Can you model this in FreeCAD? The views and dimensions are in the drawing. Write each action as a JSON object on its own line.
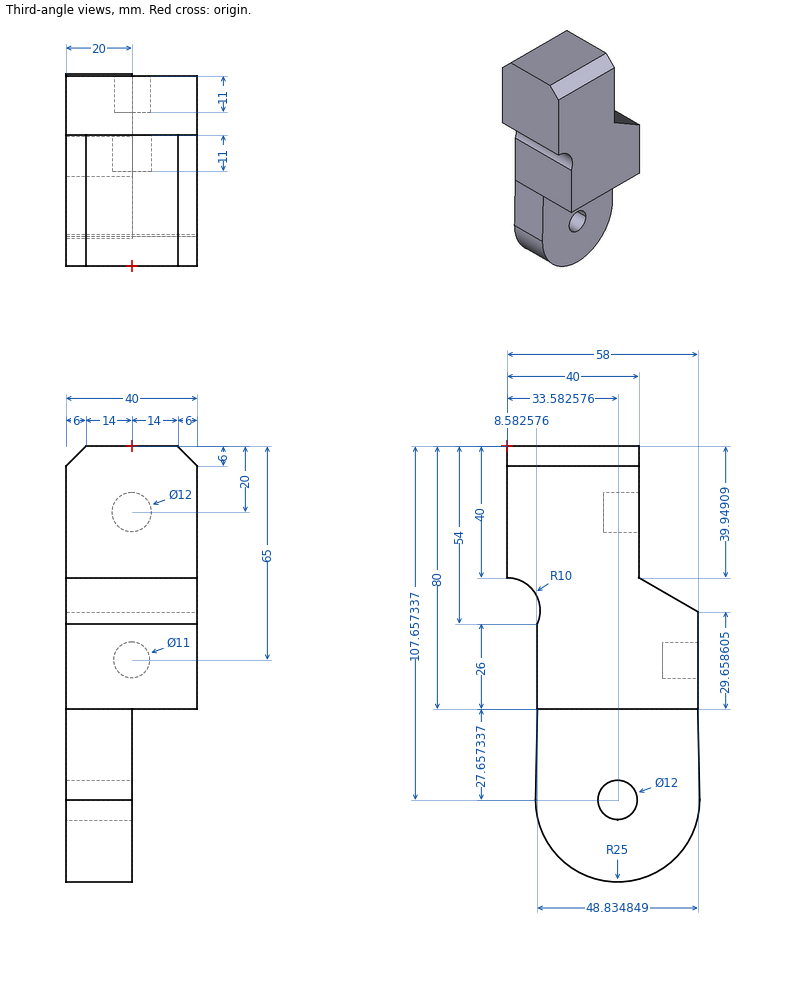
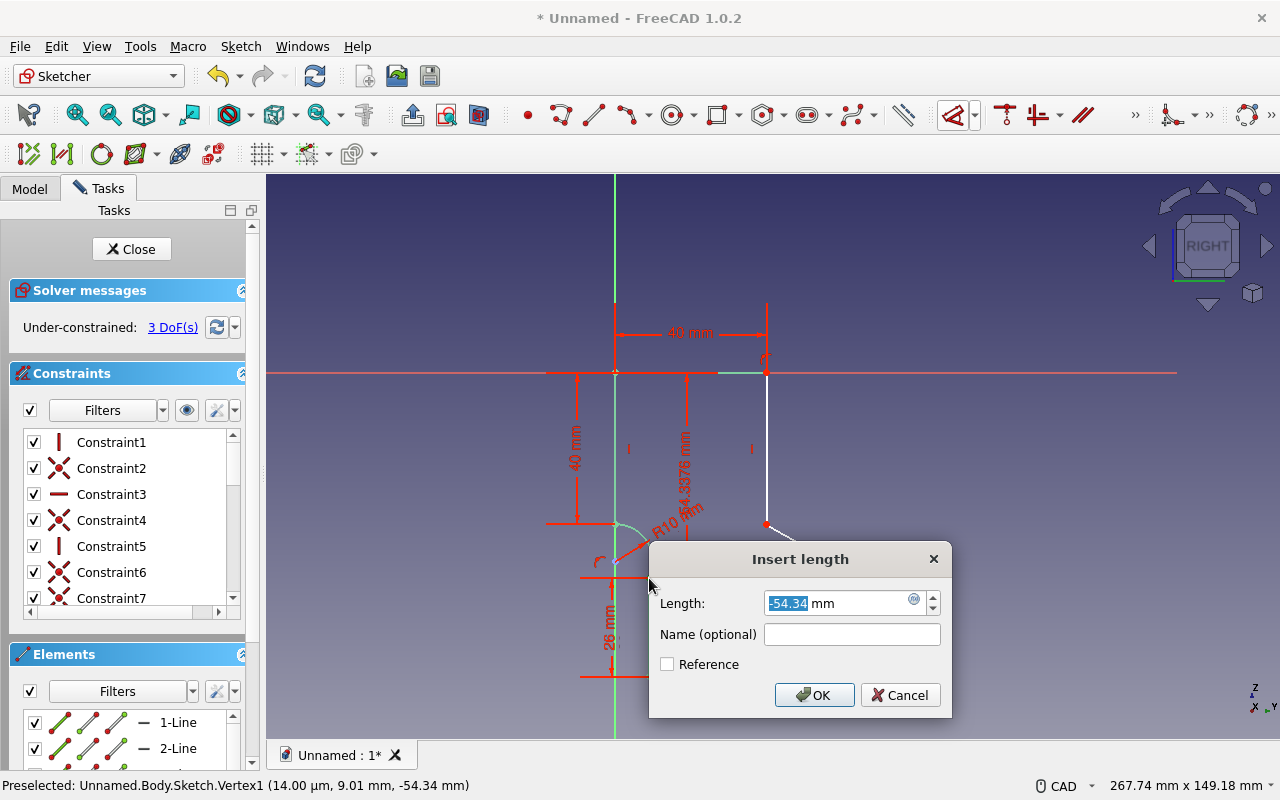
{"action": "type", "text": "-54"}
{"action": "key", "text": "Return"}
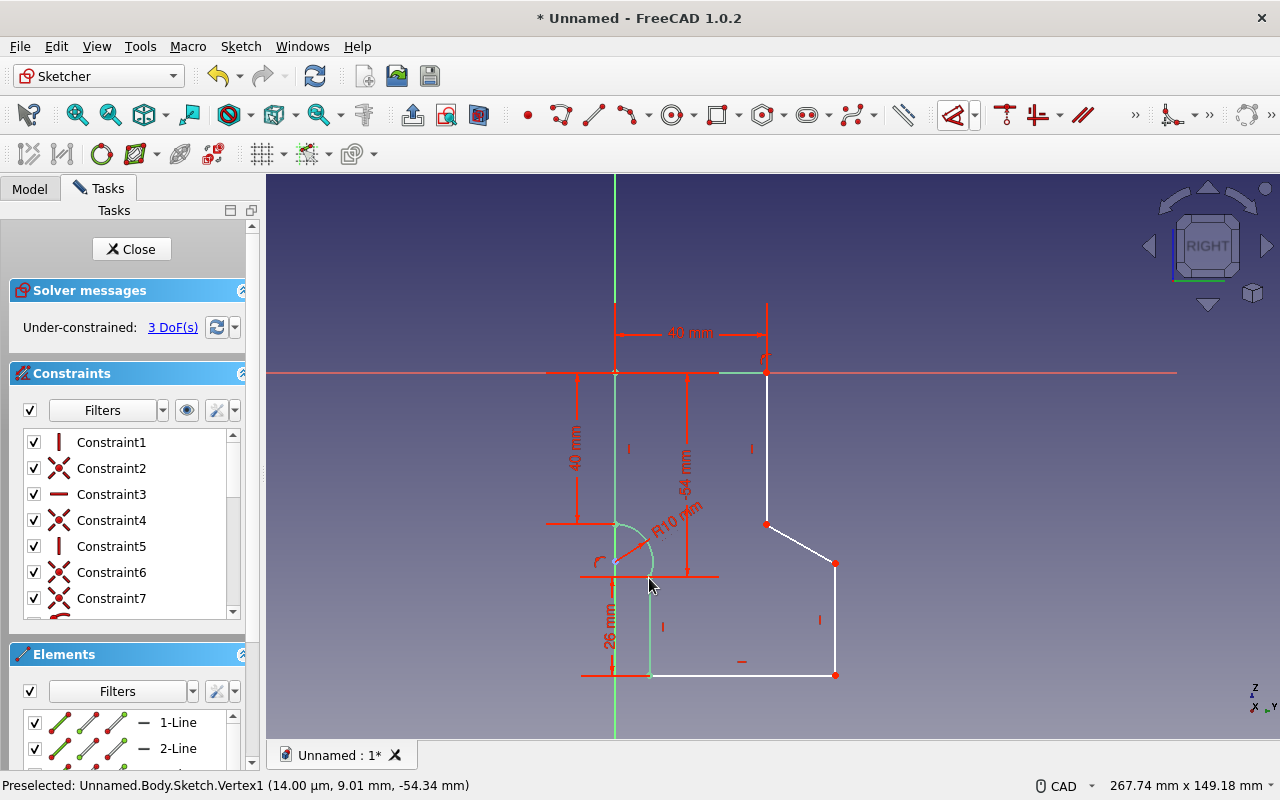
{"action": "left_click", "coordinate": [835, 676]}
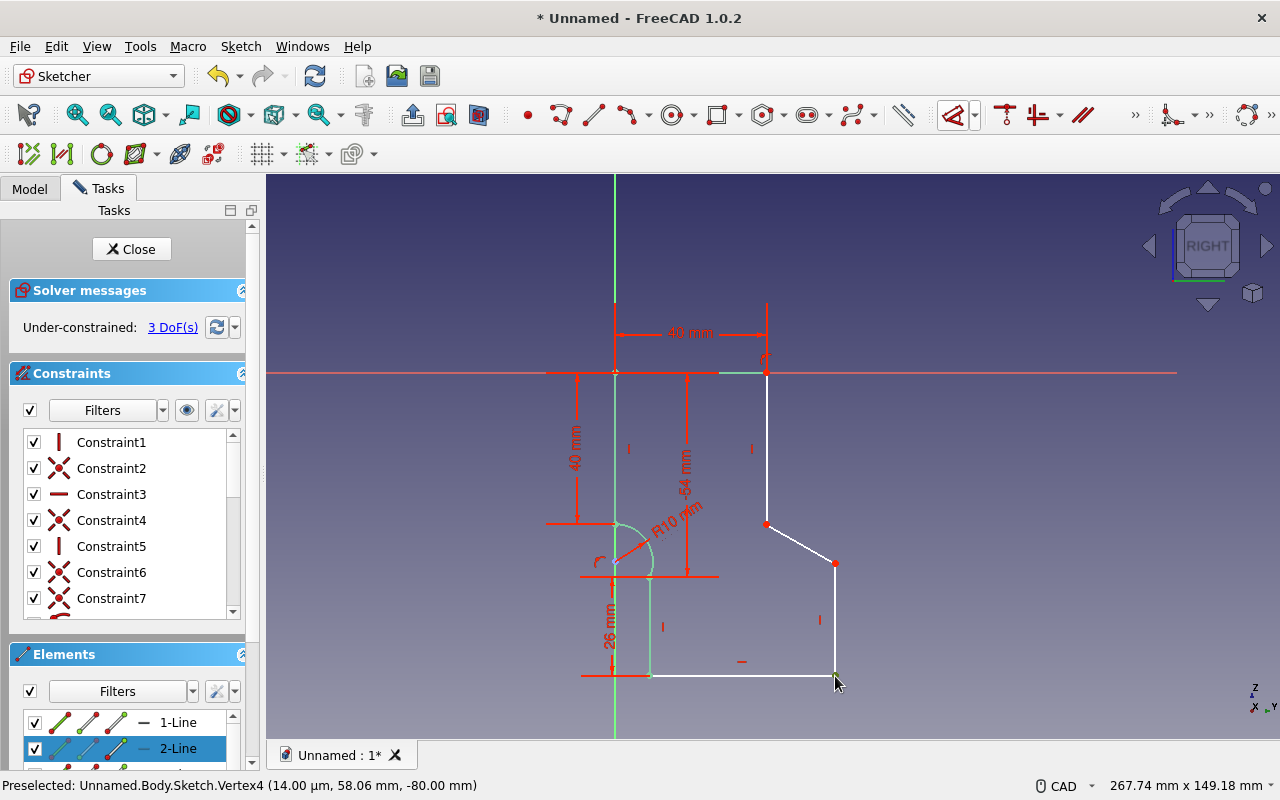
{"action": "key", "text": "l"}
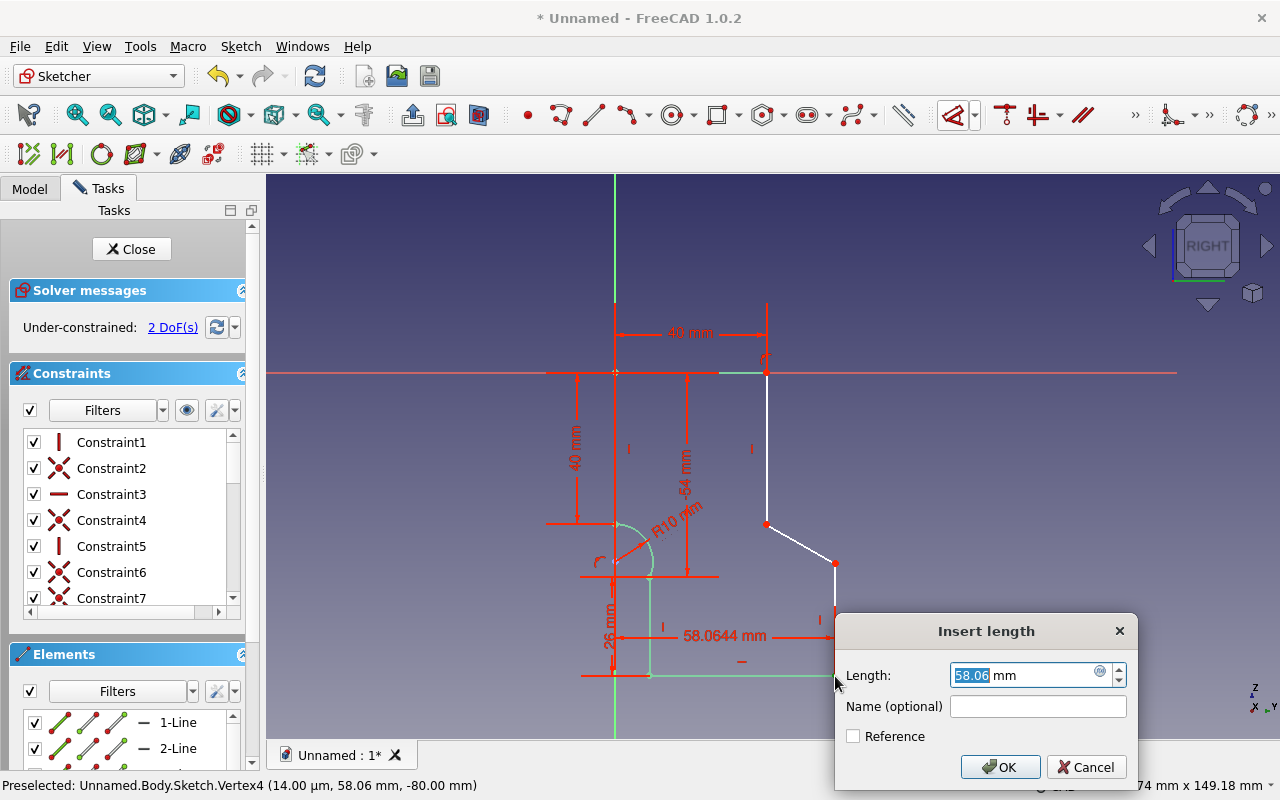
{"action": "type", "text": "58"}
{"action": "key", "text": "Return"}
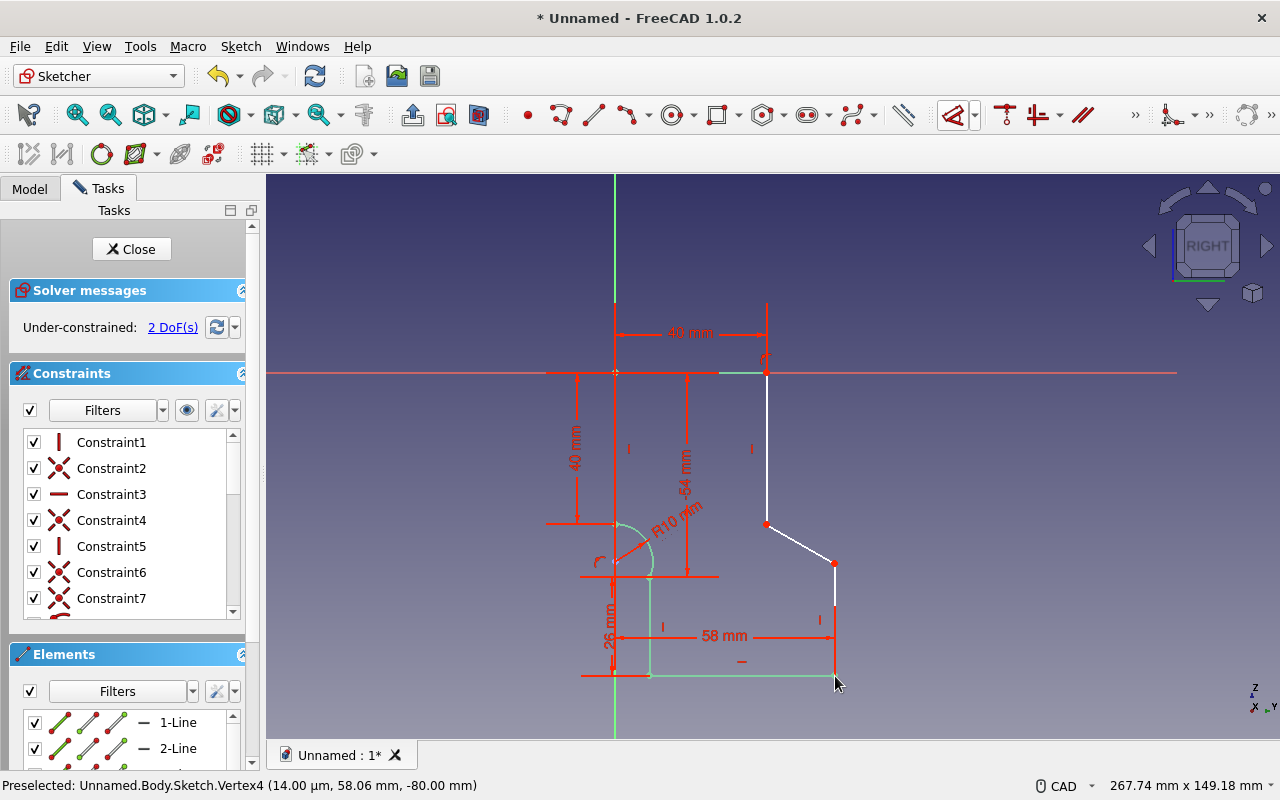
{"action": "left_click", "coordinate": [767, 479]}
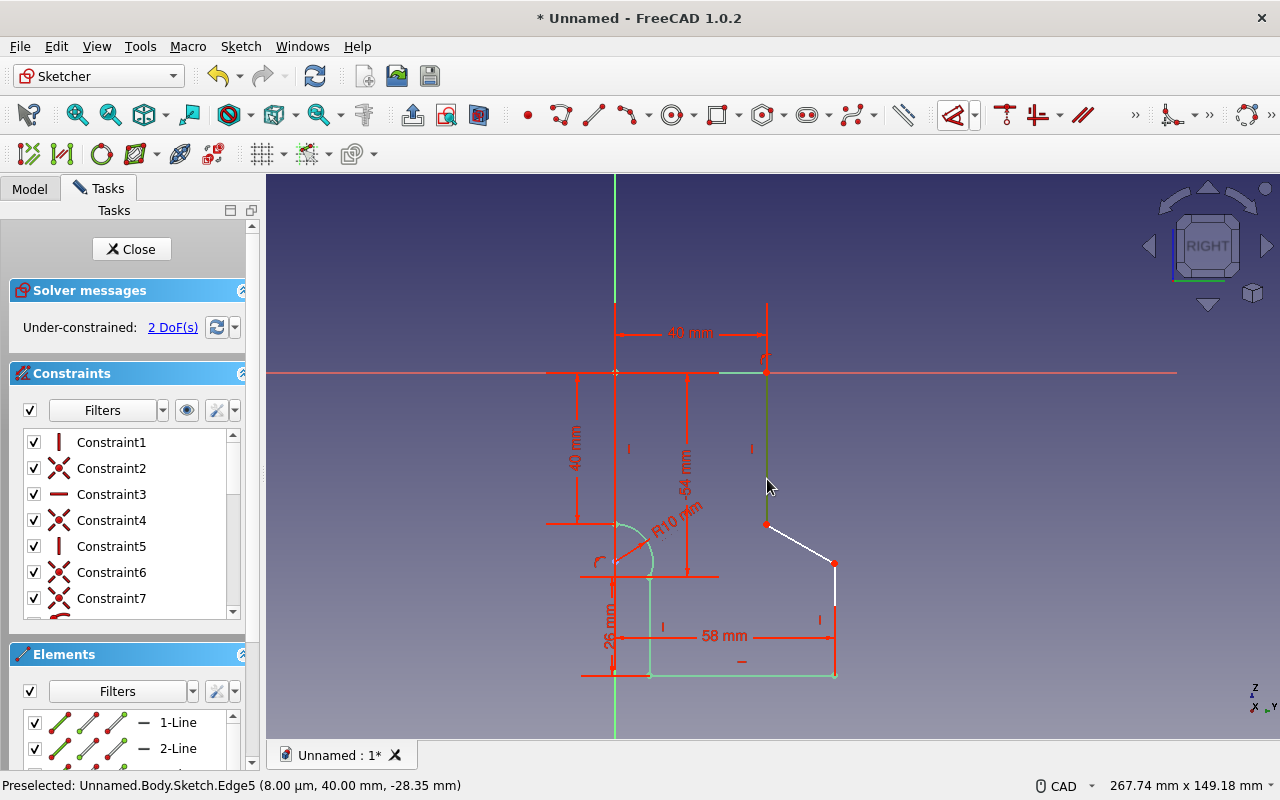
{"action": "left_click", "coordinate": [974, 116]}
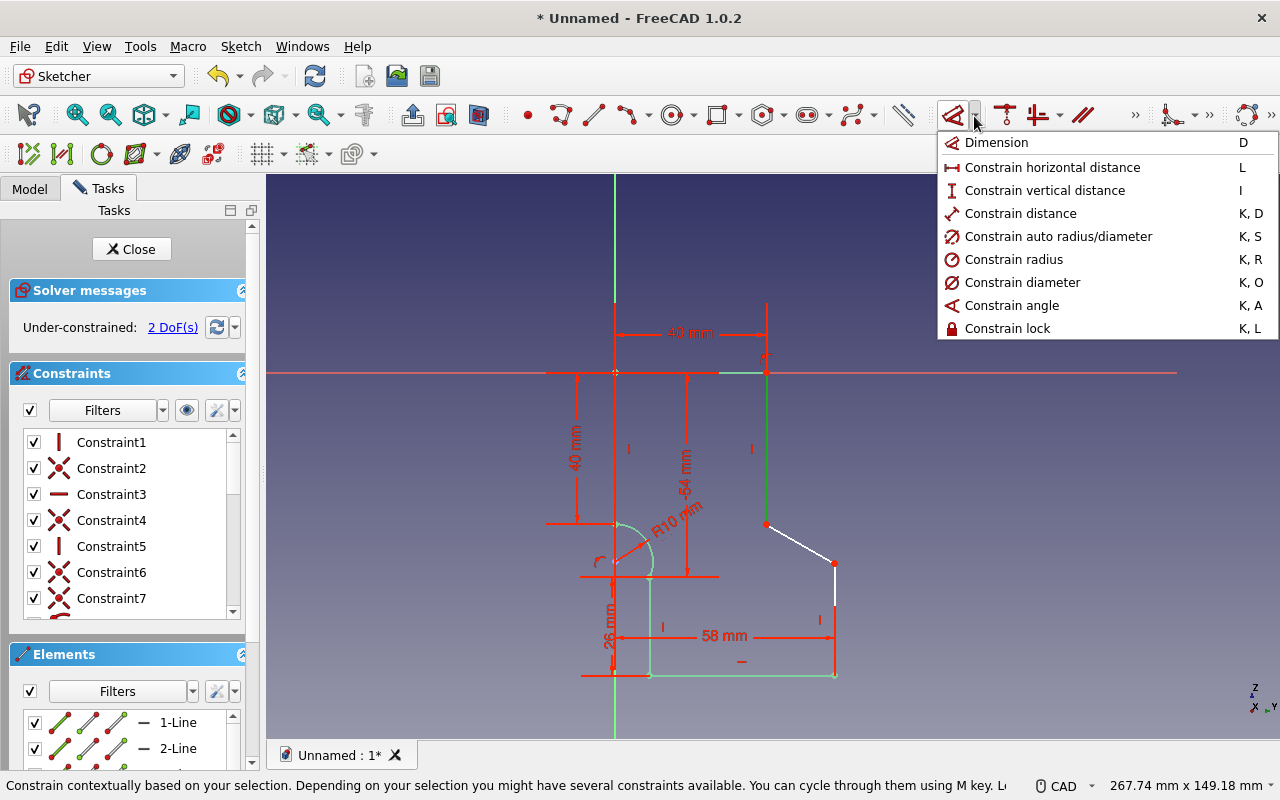
{"action": "left_click", "coordinate": [1108, 190]}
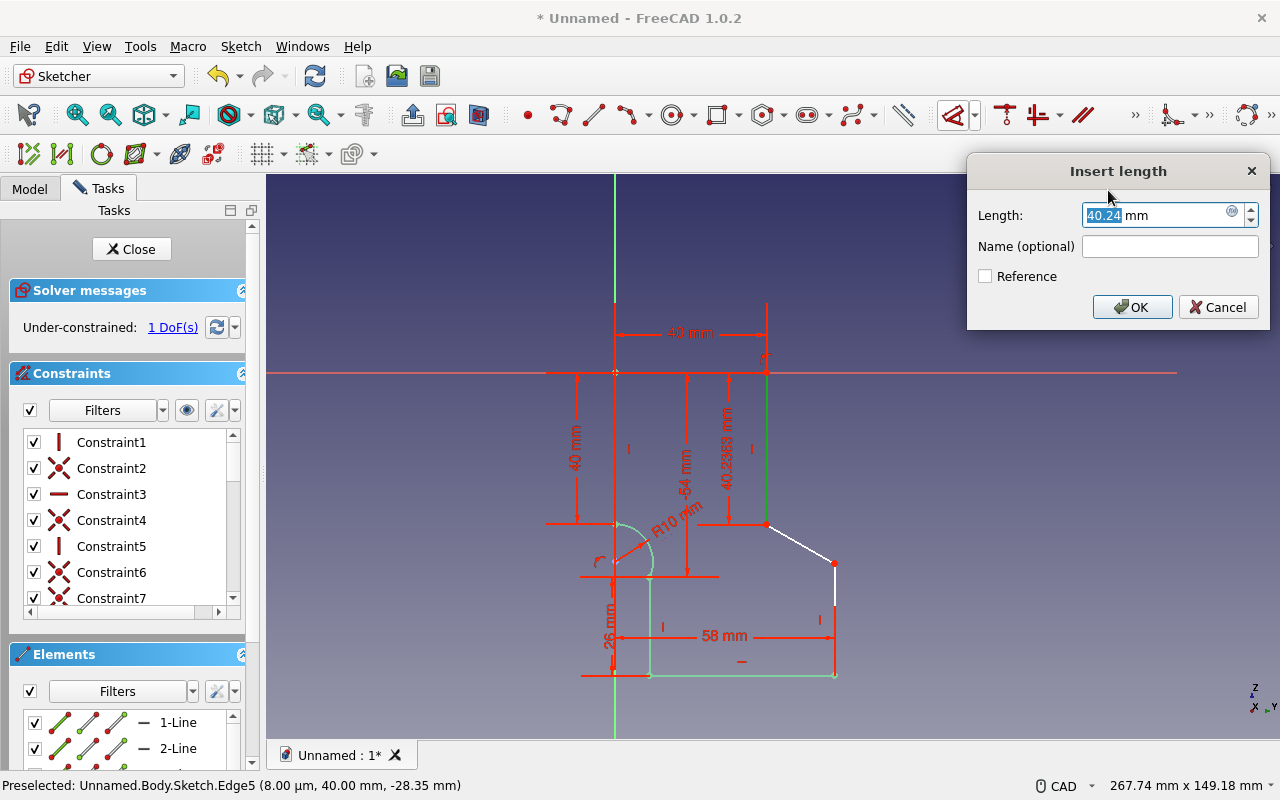
{"action": "type", "text": "39.94909"}
{"action": "key", "text": "Return"}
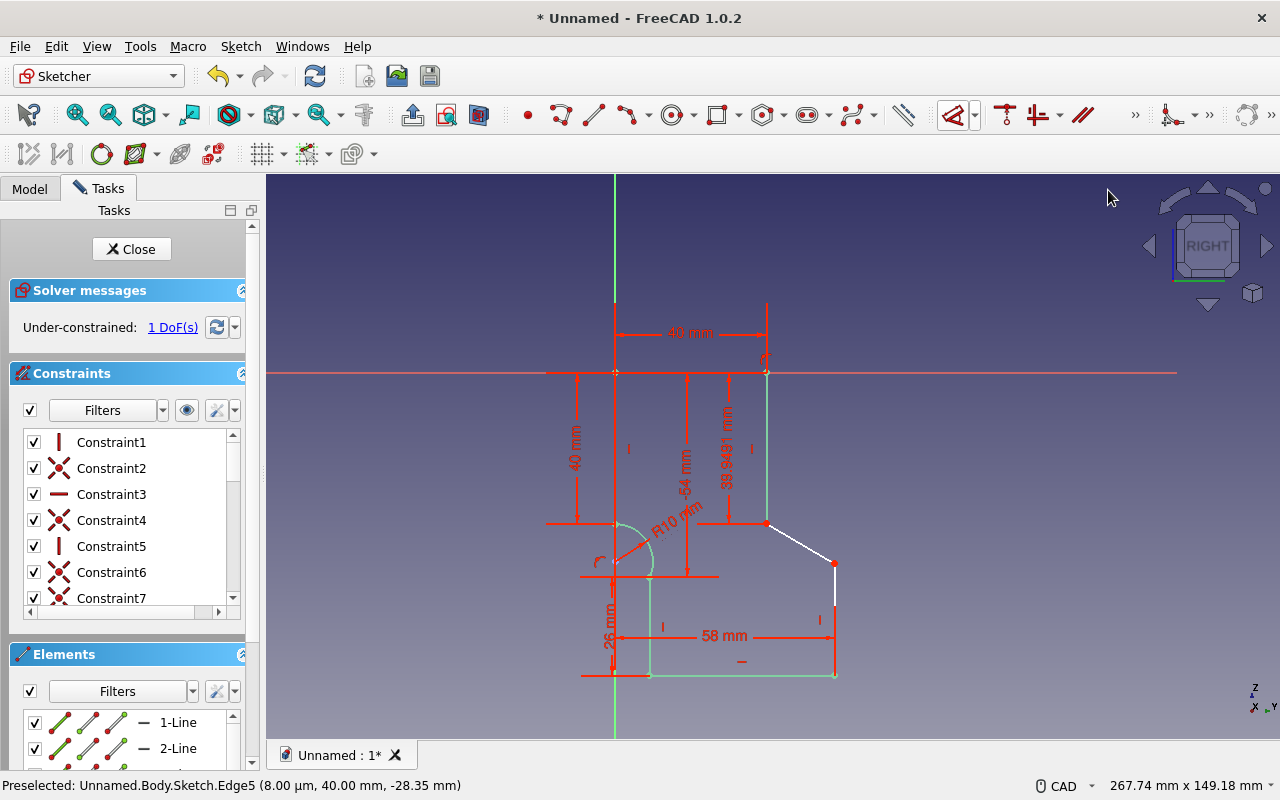
{"action": "left_click", "coordinate": [835, 642]}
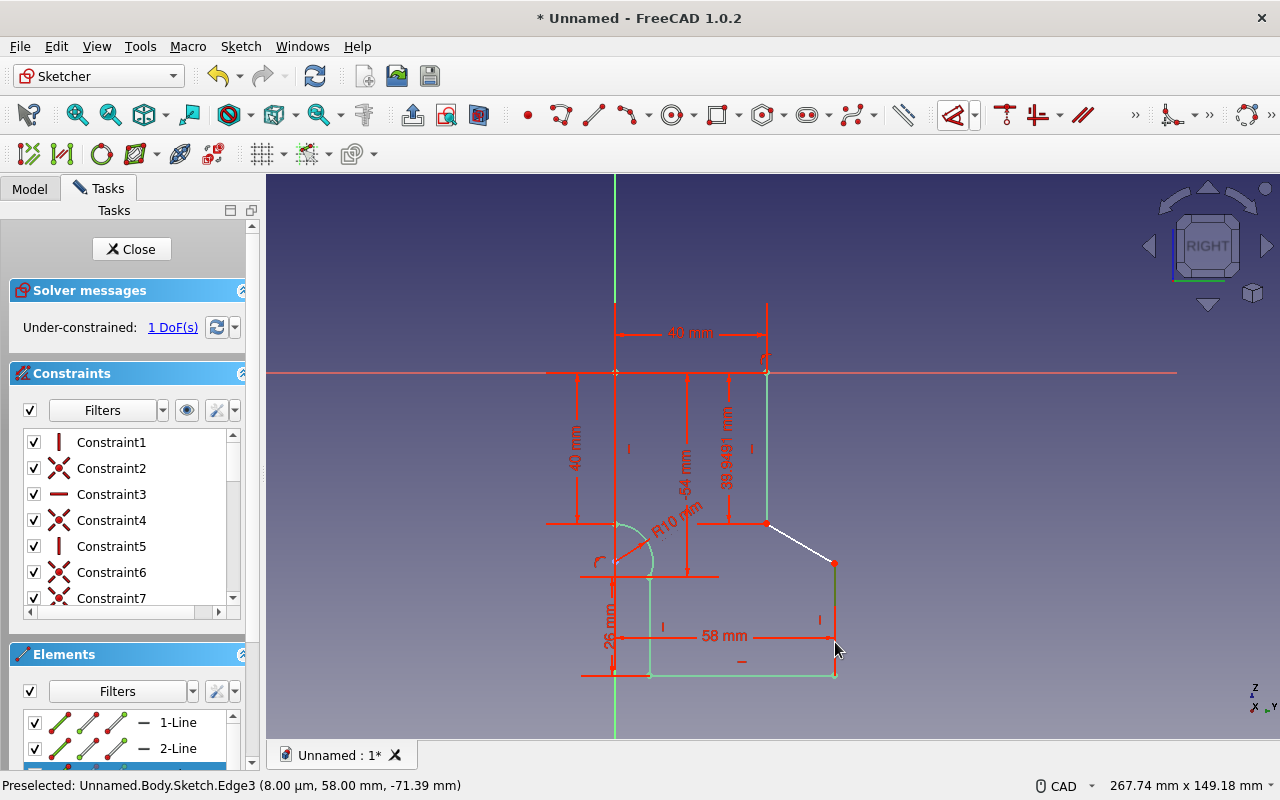
{"action": "key", "text": "i"}